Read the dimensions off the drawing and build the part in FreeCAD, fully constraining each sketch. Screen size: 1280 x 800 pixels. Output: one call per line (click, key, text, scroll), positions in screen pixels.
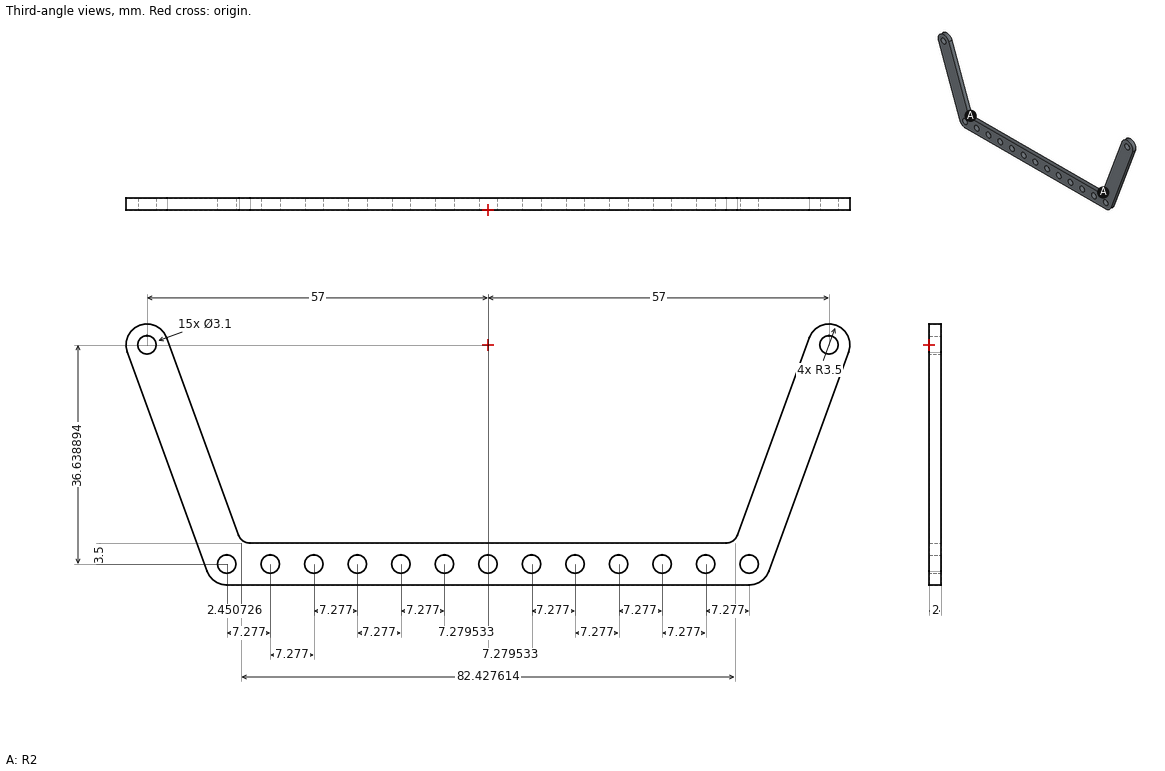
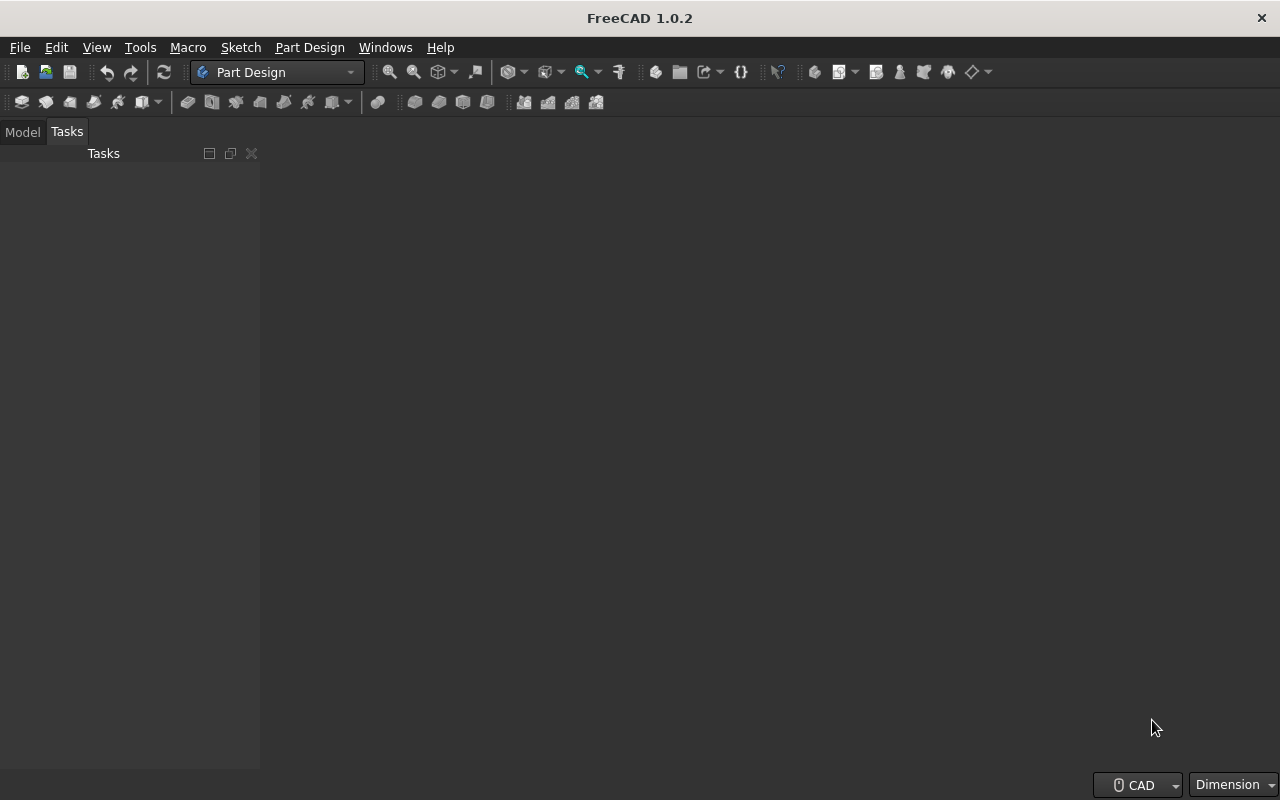
click(22, 72)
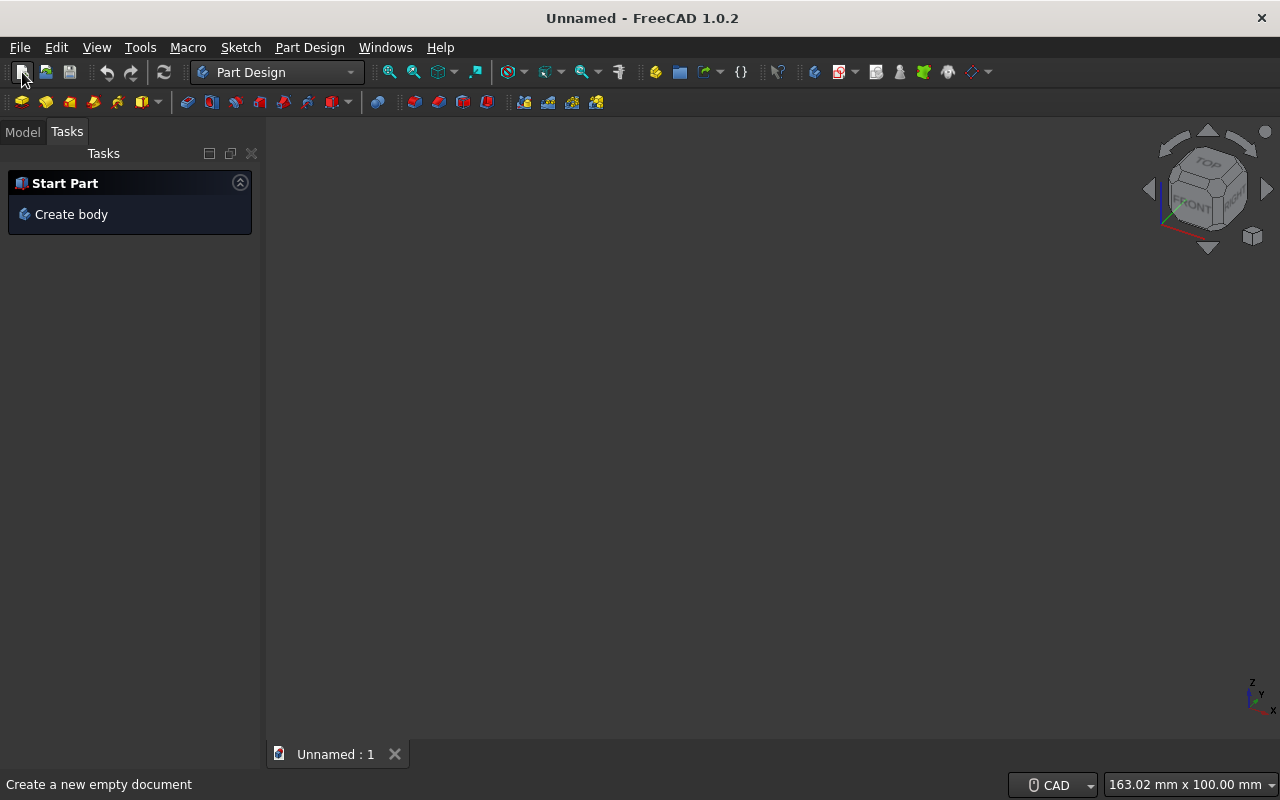
click(840, 72)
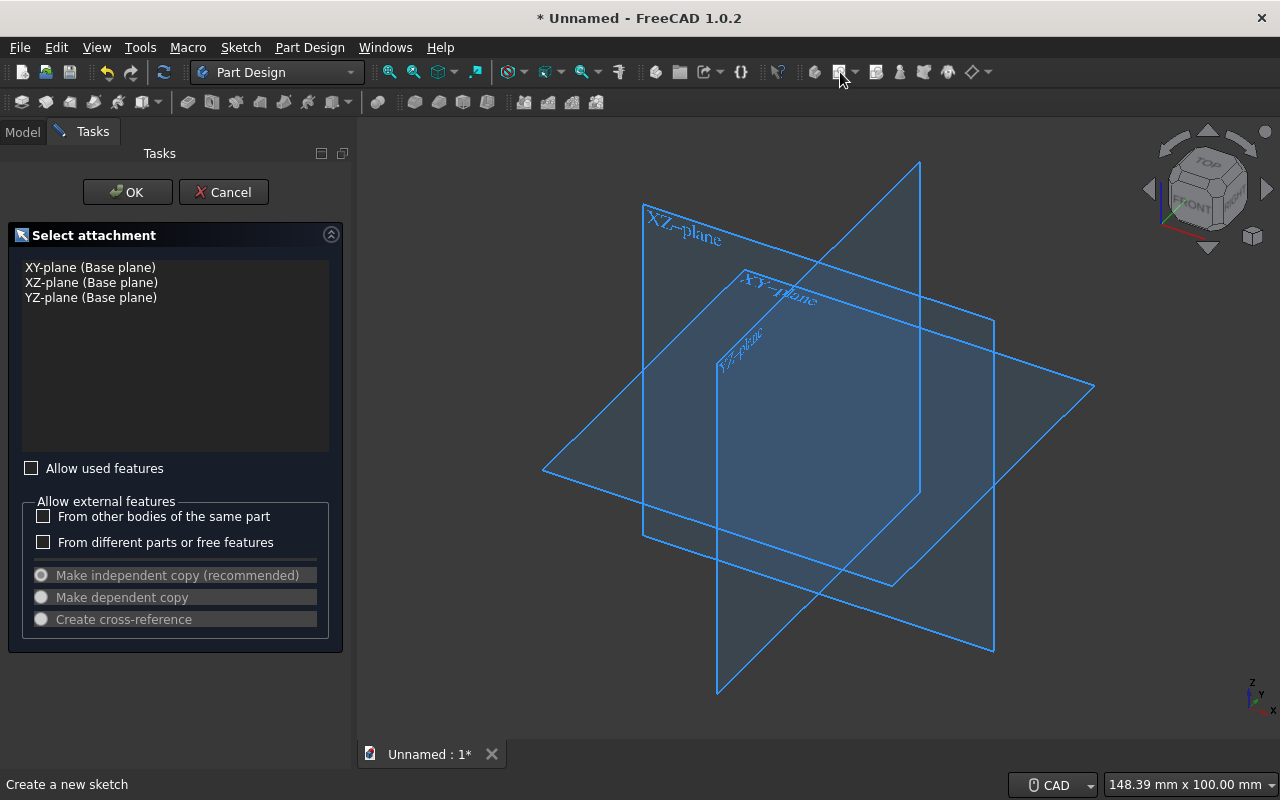
click(82, 282)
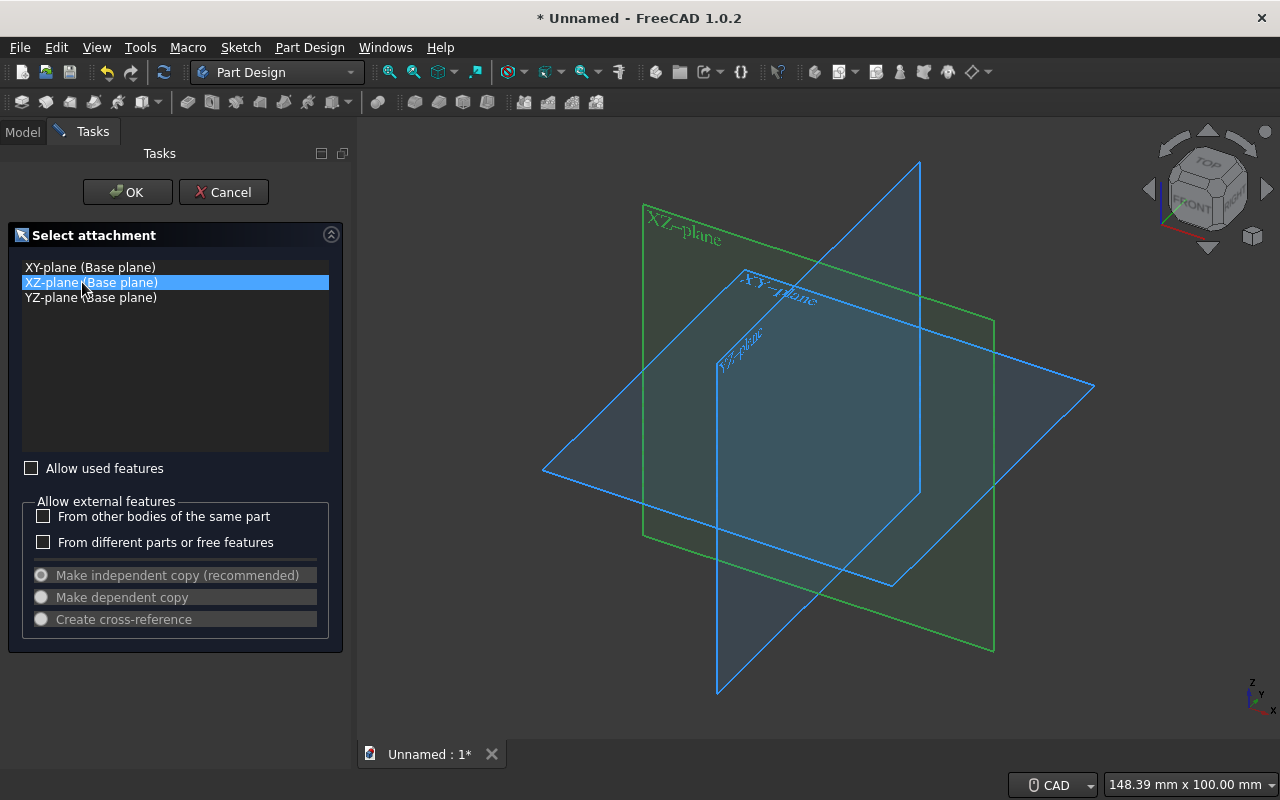
click(128, 192)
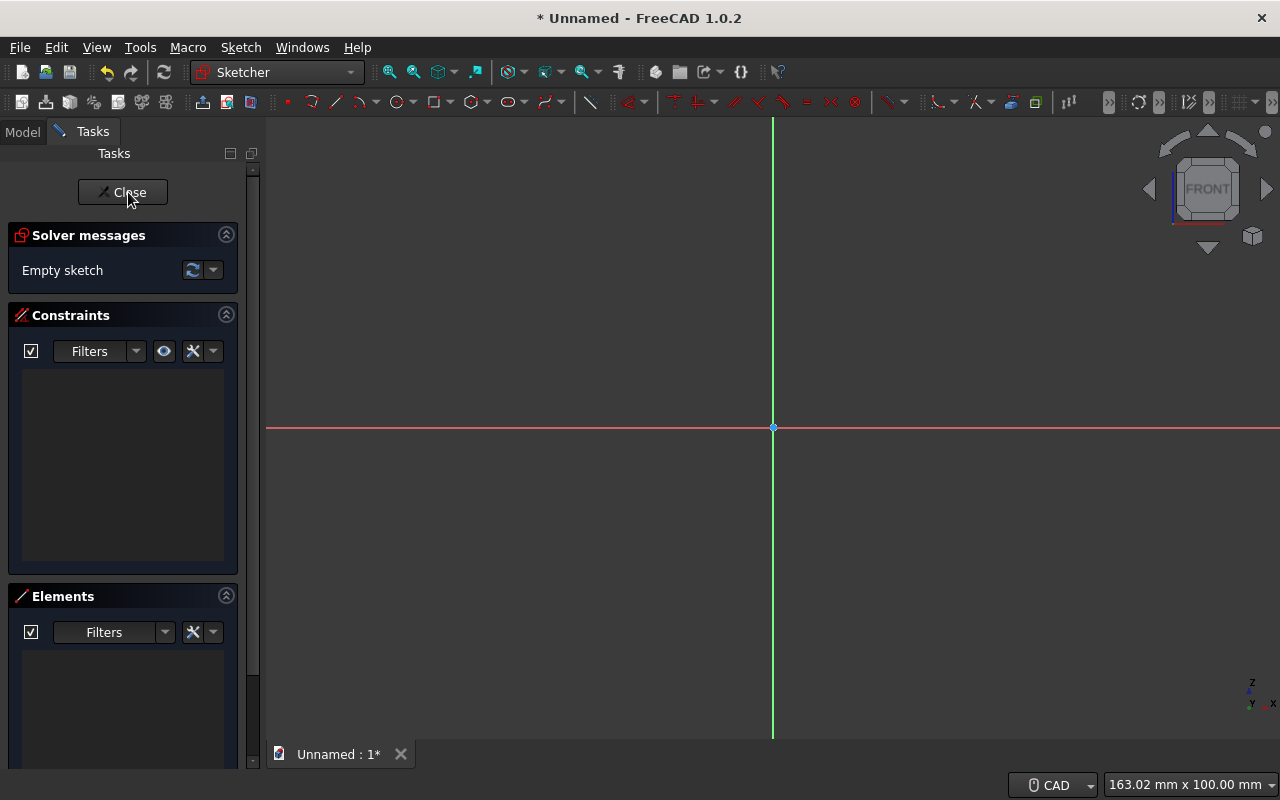
scroll(395, 145, down, 1)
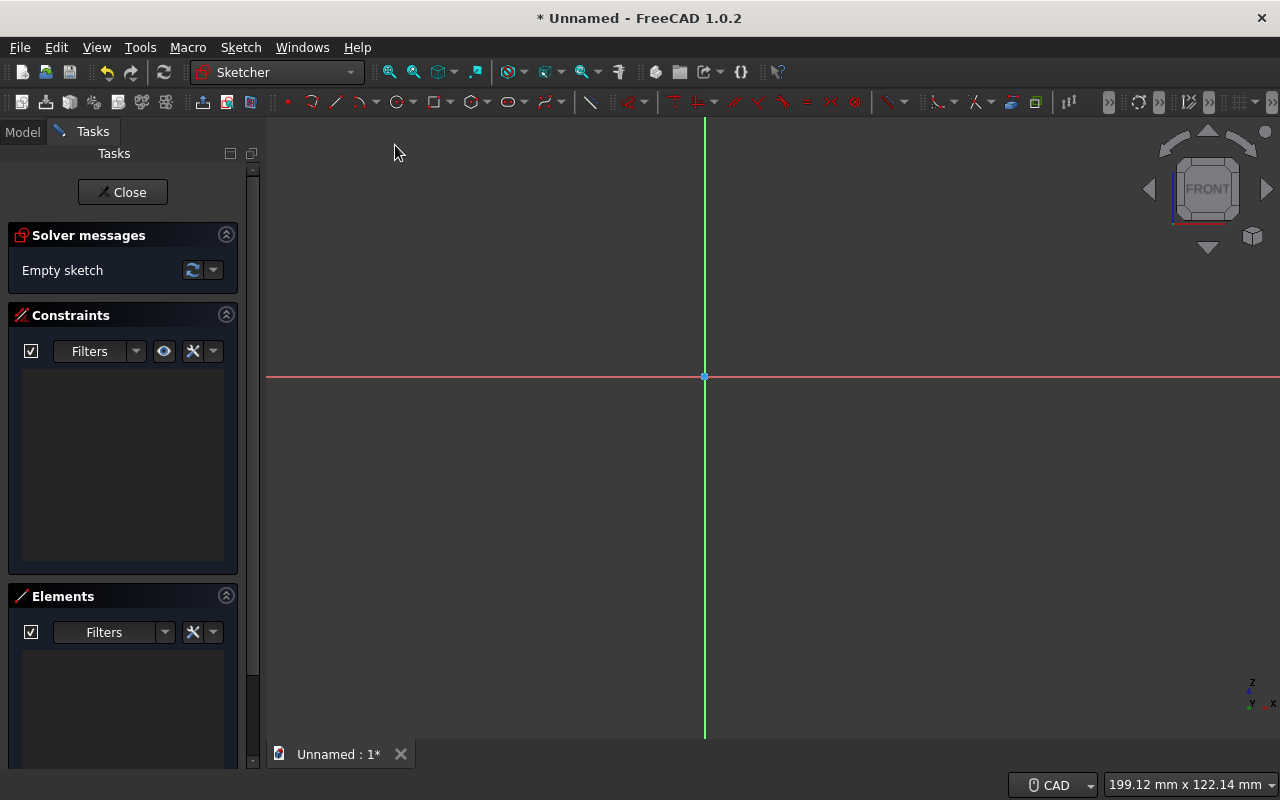
key(g)
key(l)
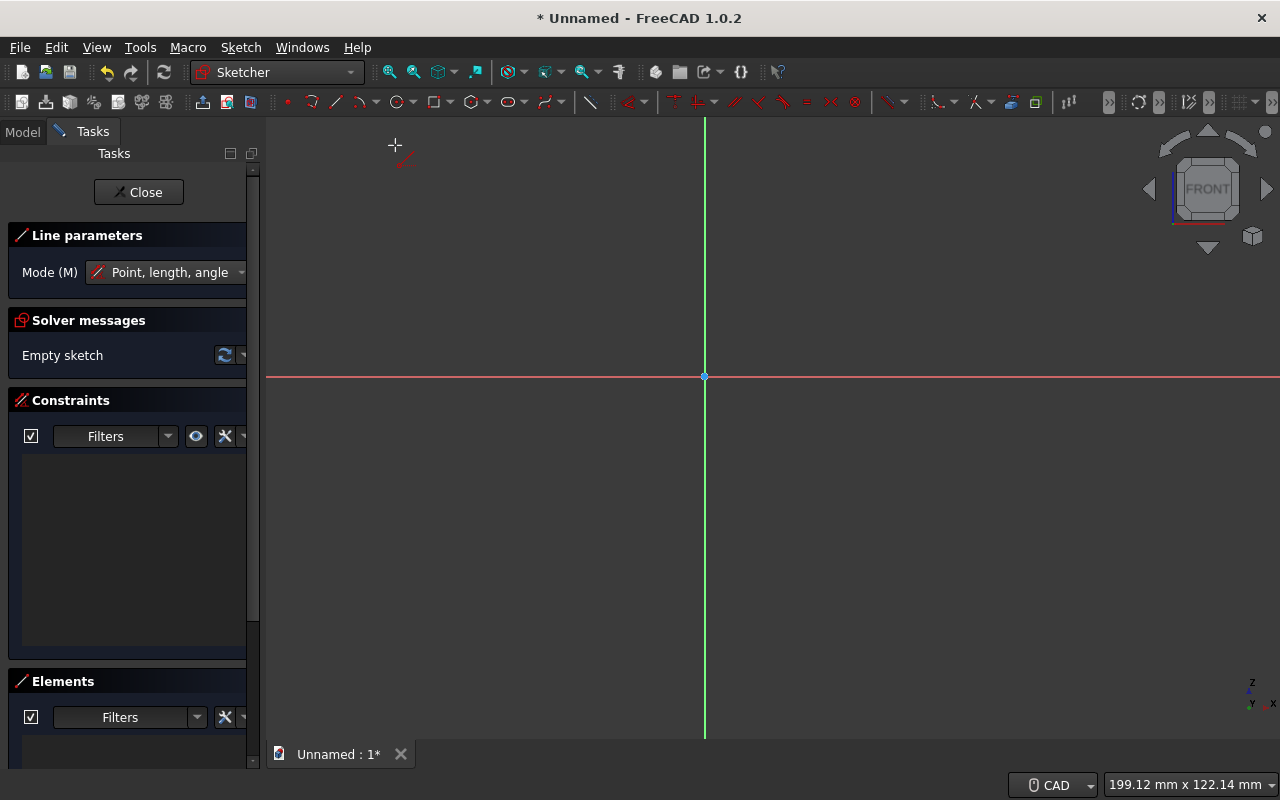
scroll(1012, 383, up, 5)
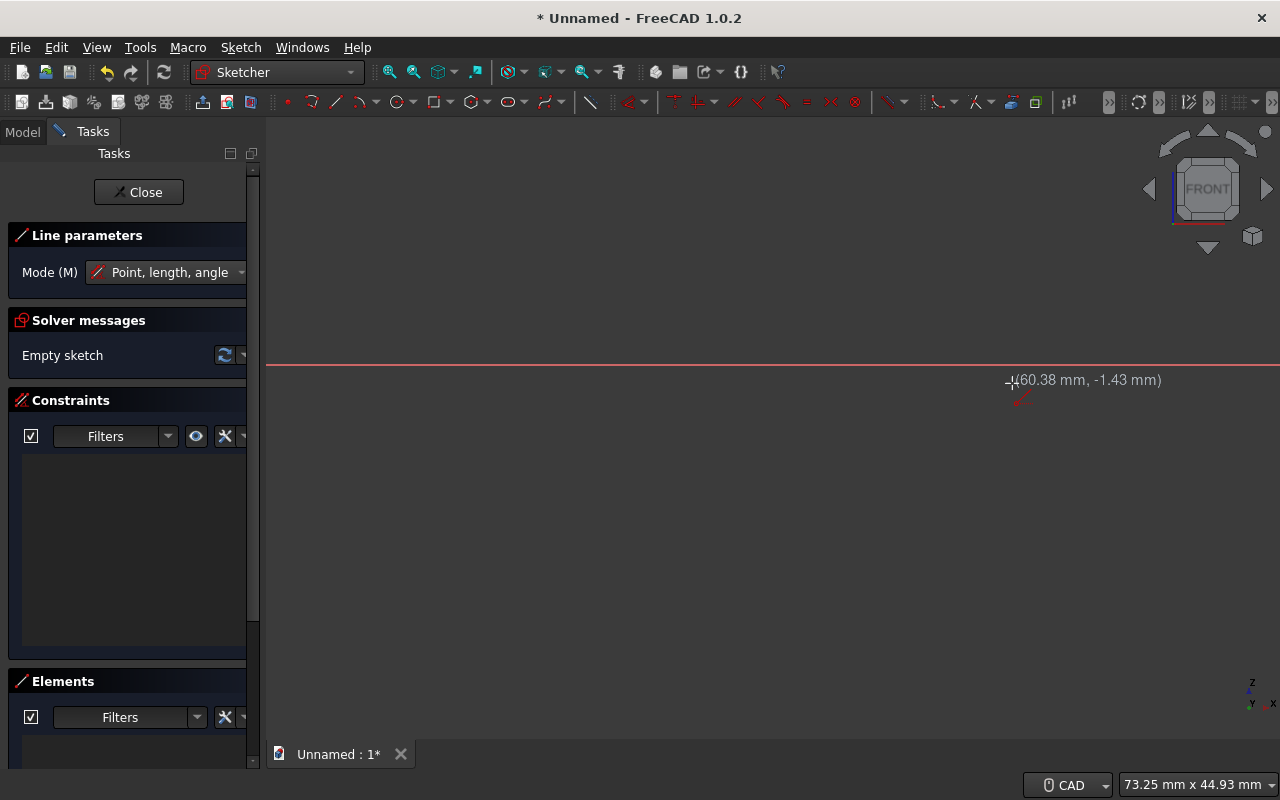
click(1009, 382)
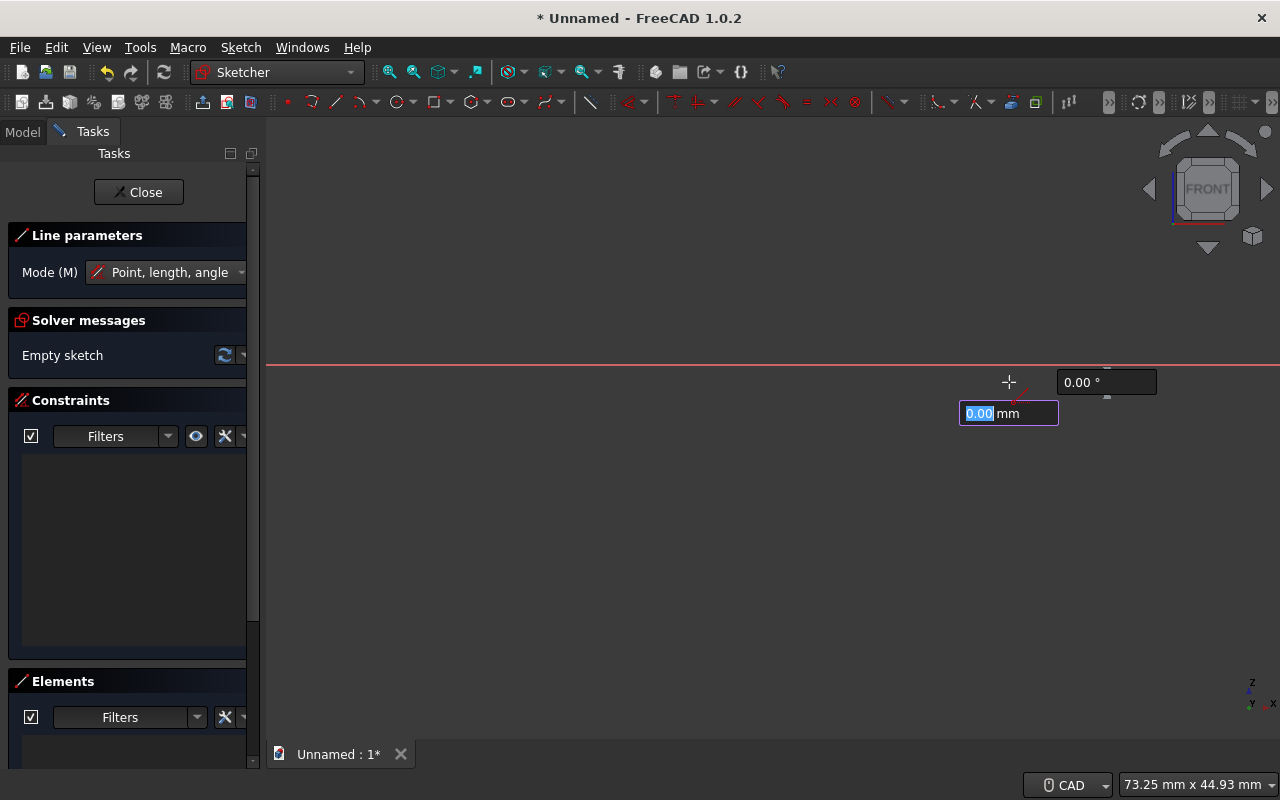
scroll(1013, 316, down, 5)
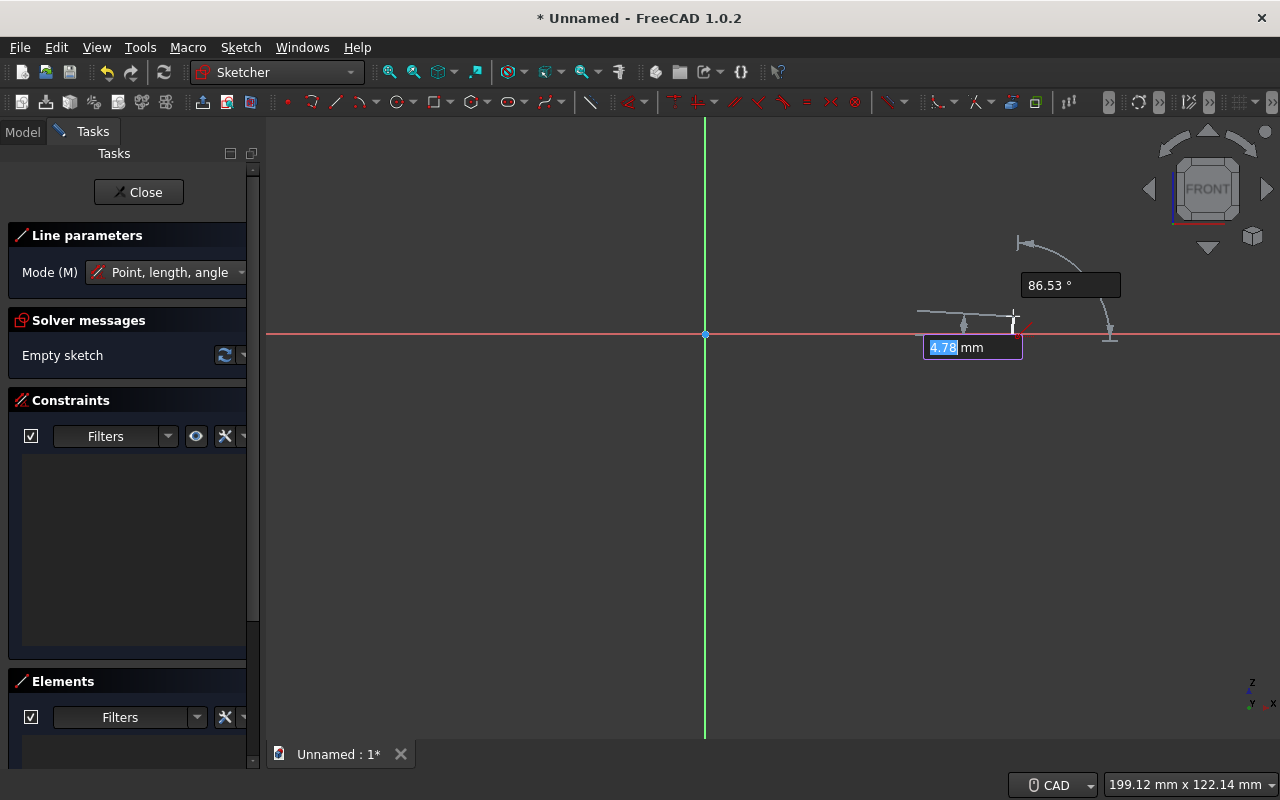
click(944, 527)